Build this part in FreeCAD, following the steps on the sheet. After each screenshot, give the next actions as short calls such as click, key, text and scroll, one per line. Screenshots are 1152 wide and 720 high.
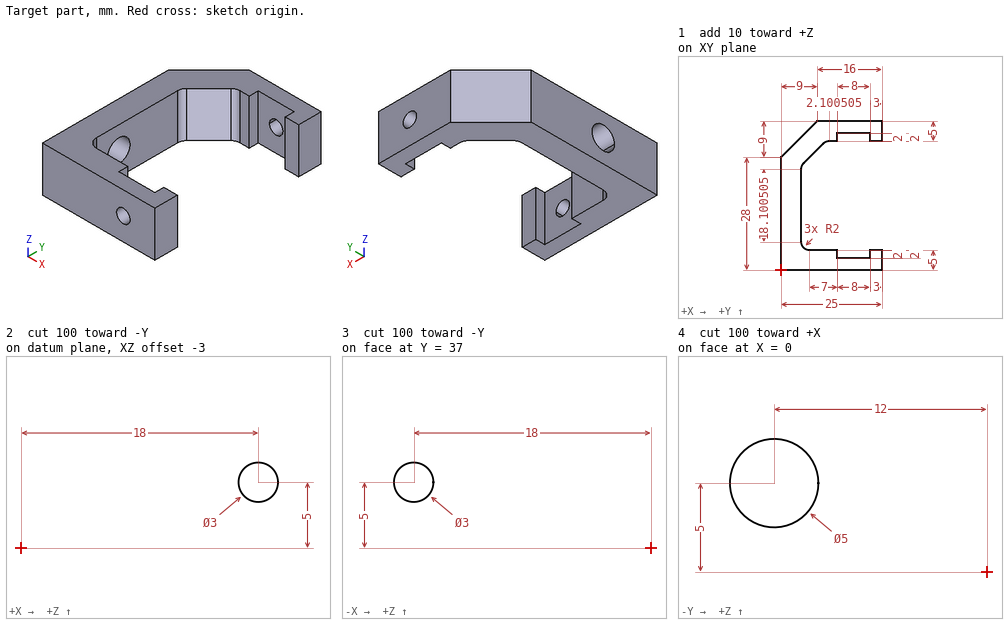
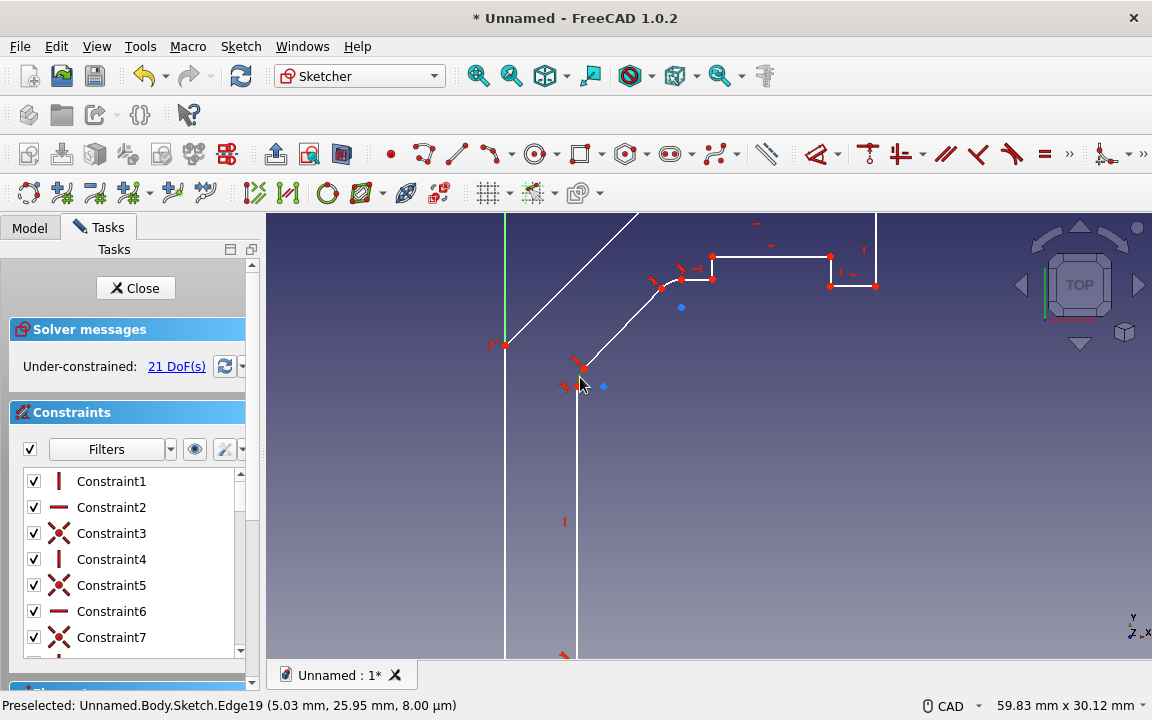
scroll(632, 324, up, 7)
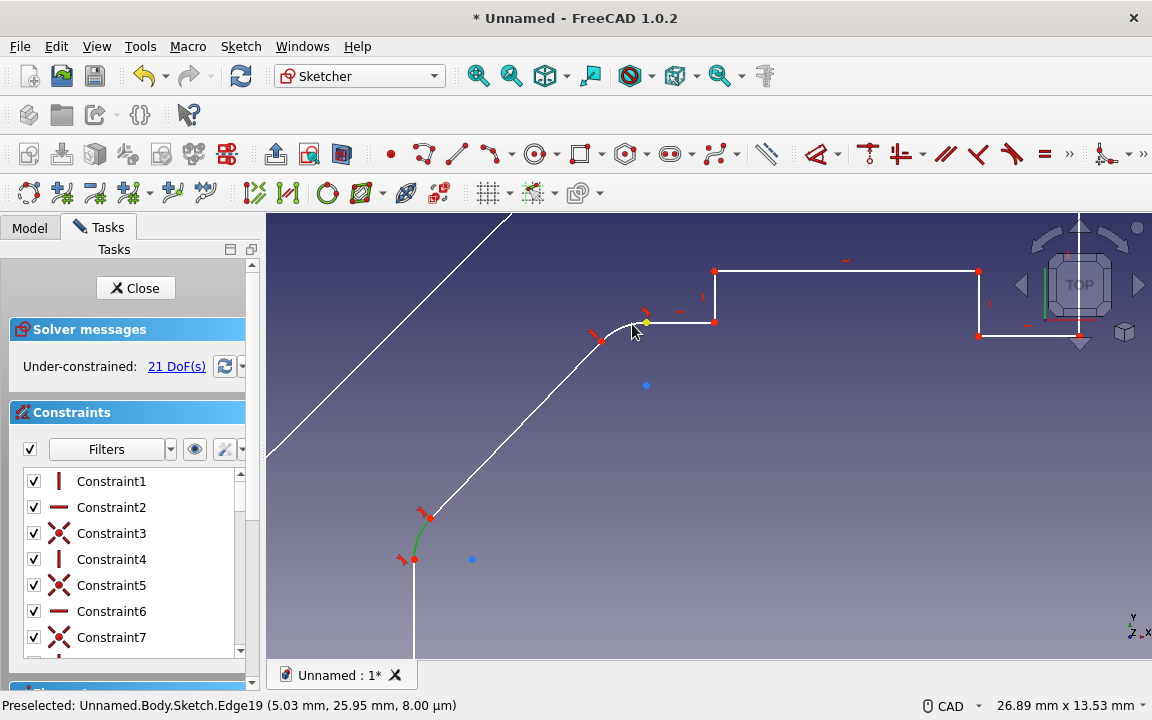
click(631, 324)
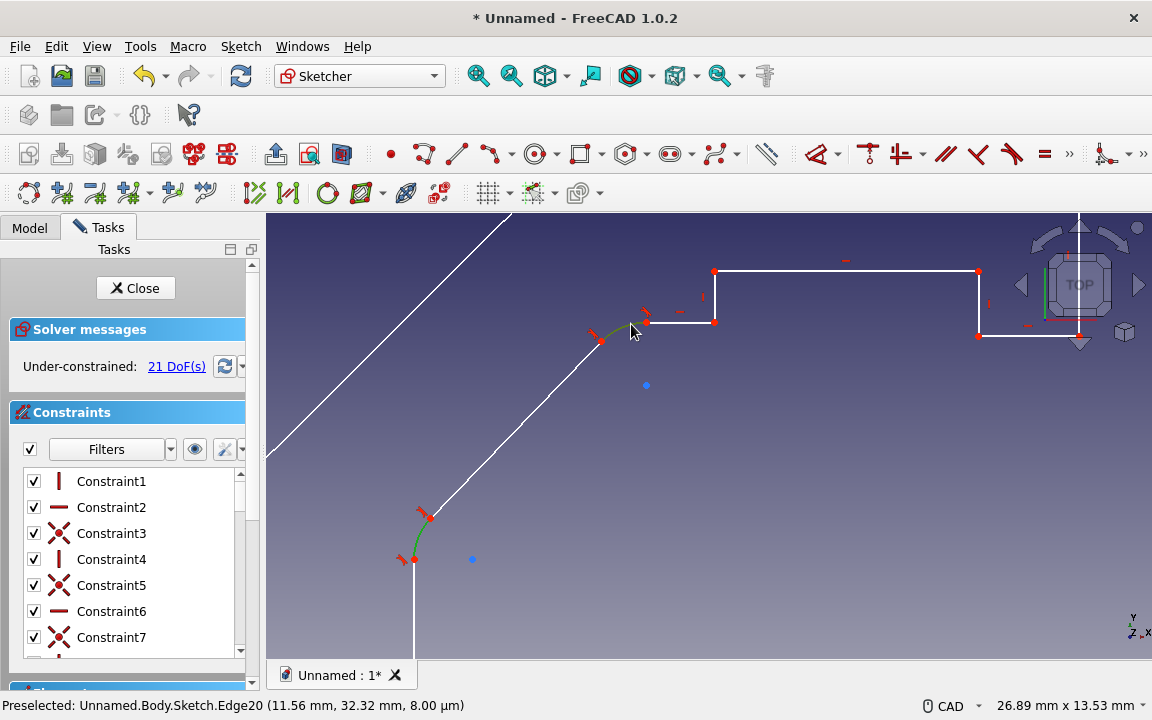
scroll(632, 324, down, 7)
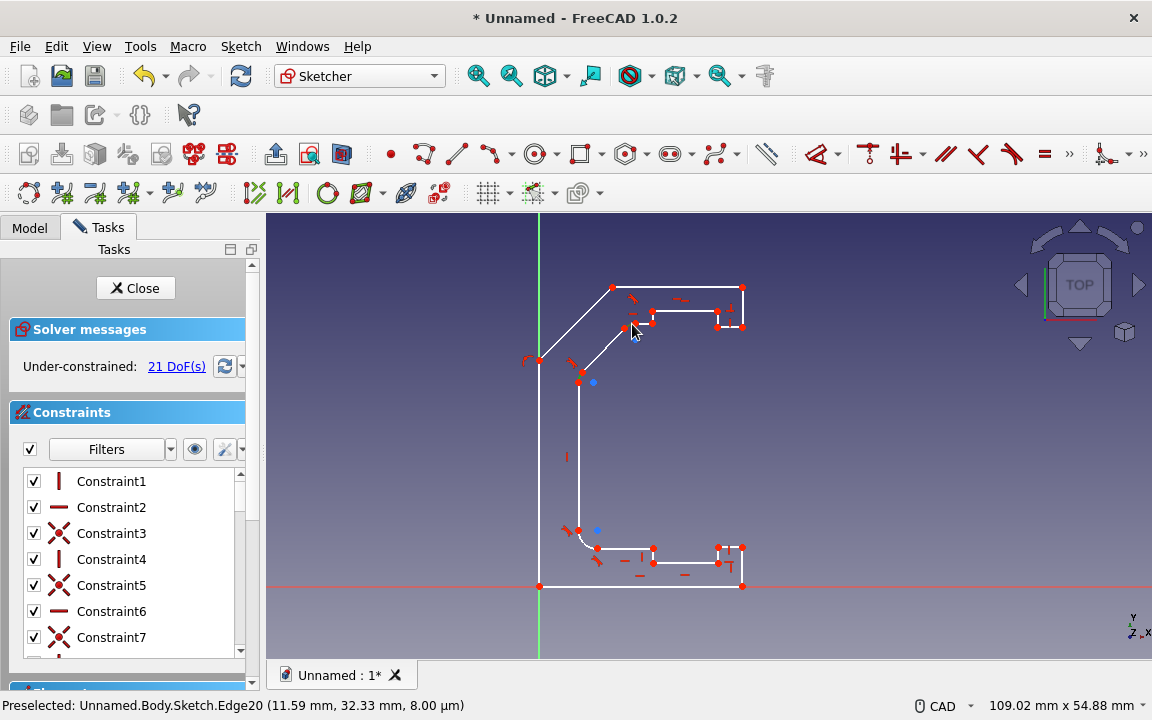
scroll(581, 539, up, 3)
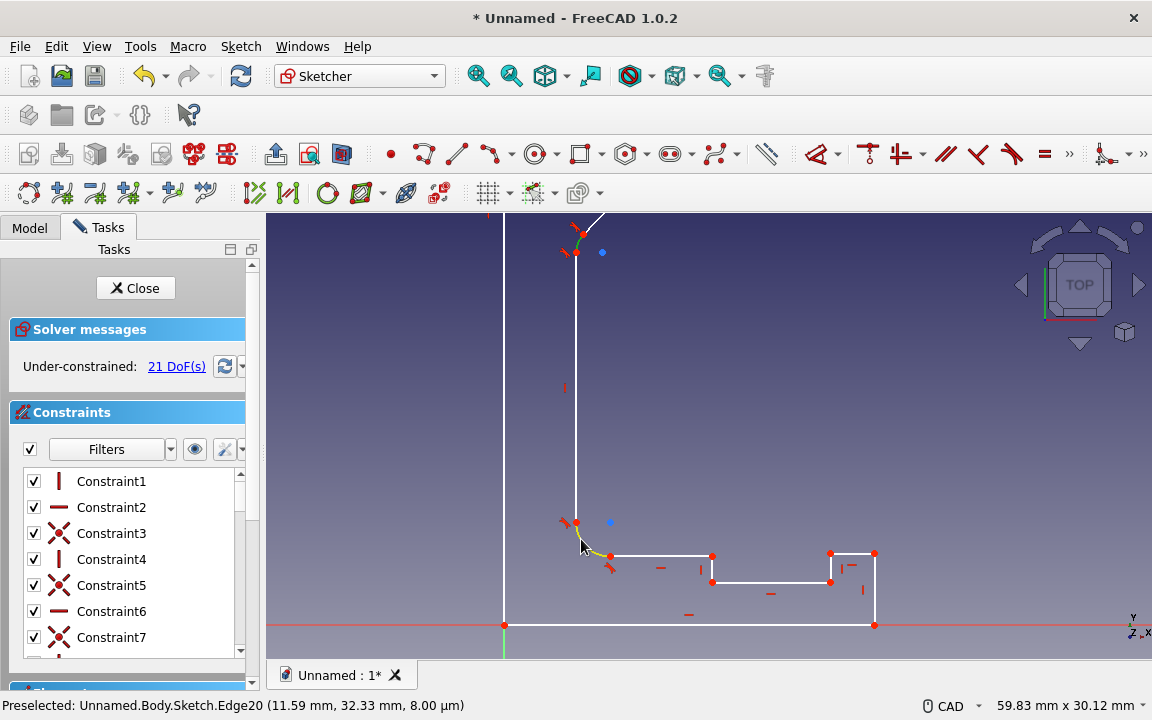
click(580, 538)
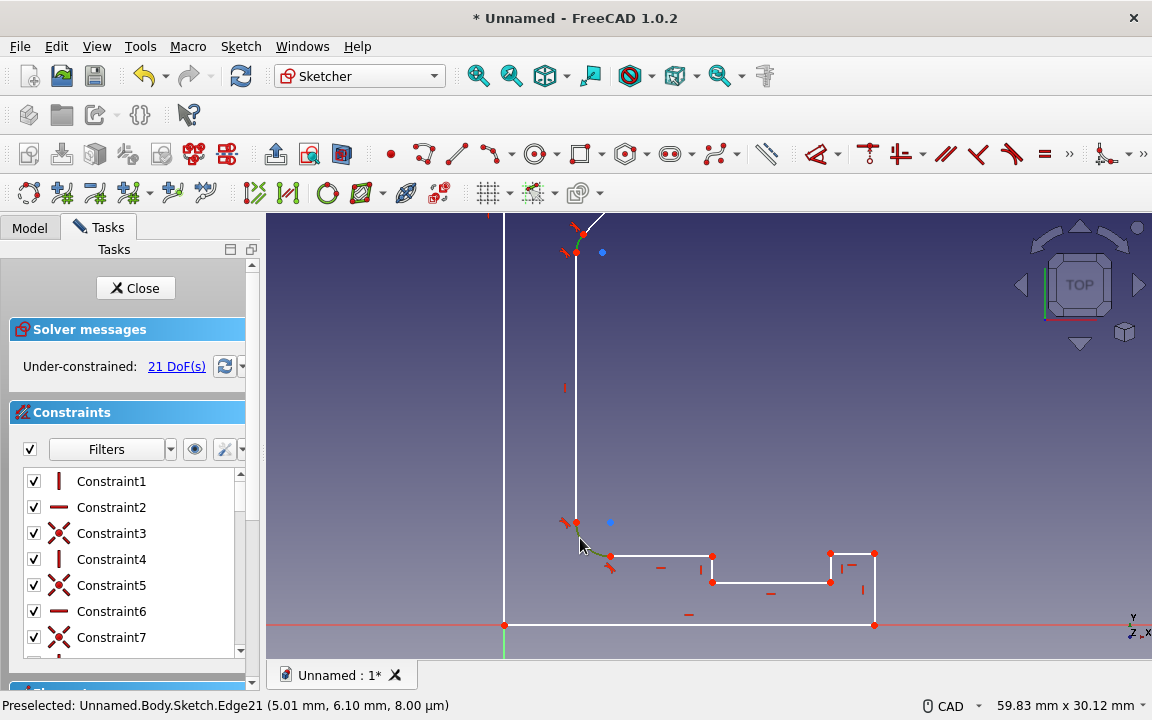
key(e)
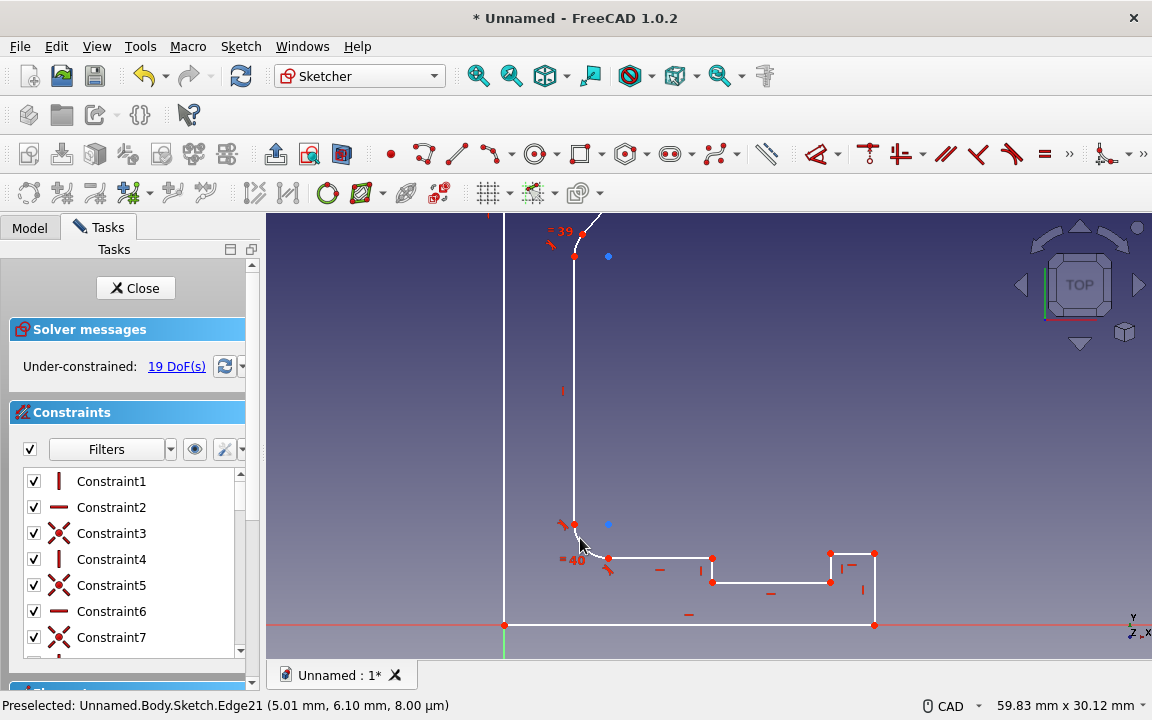
key(d)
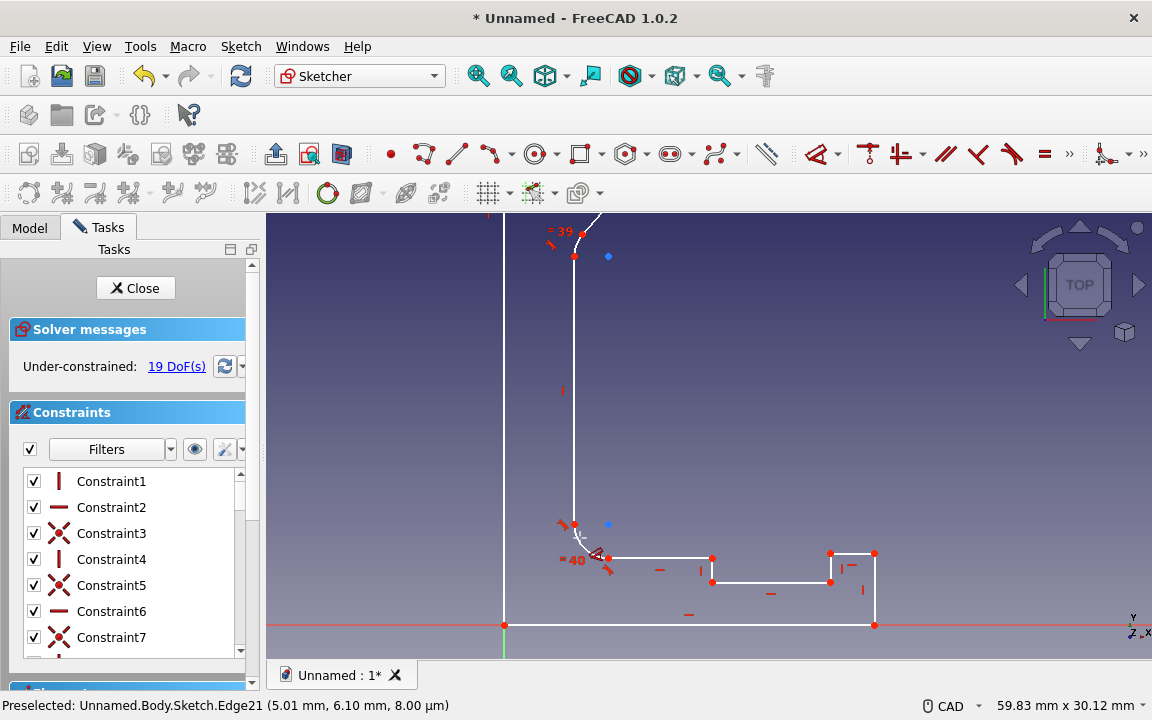
scroll(577, 245, up, 2)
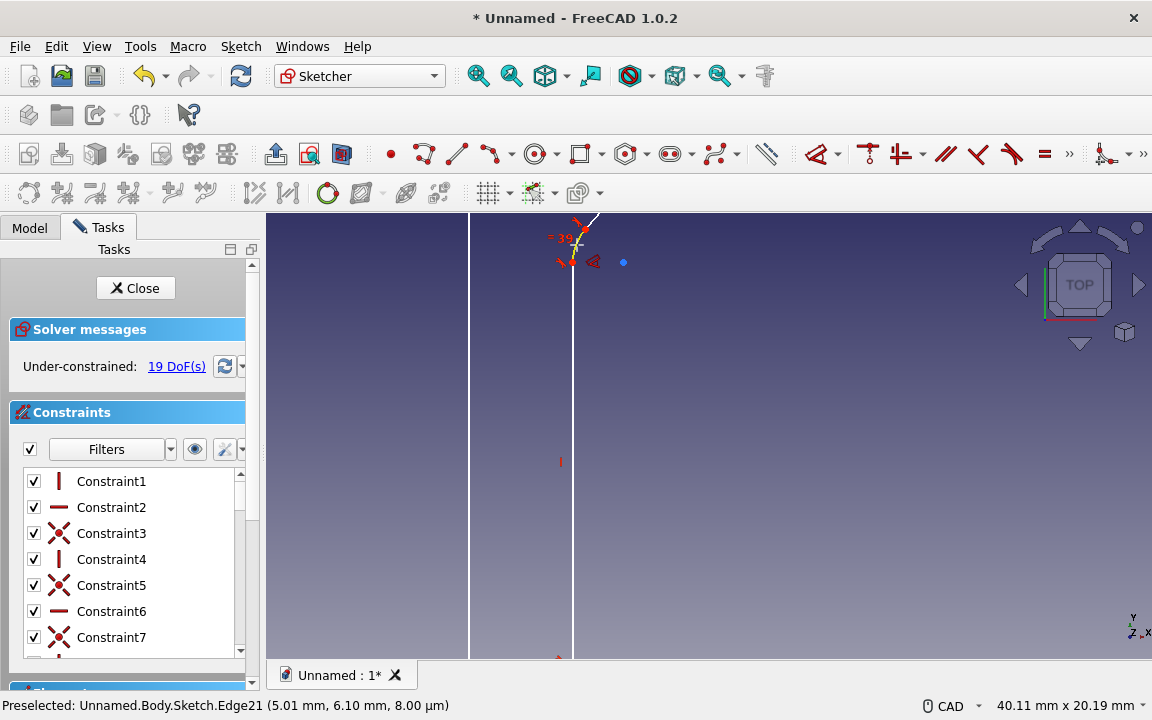
click(576, 245)
click(542, 275)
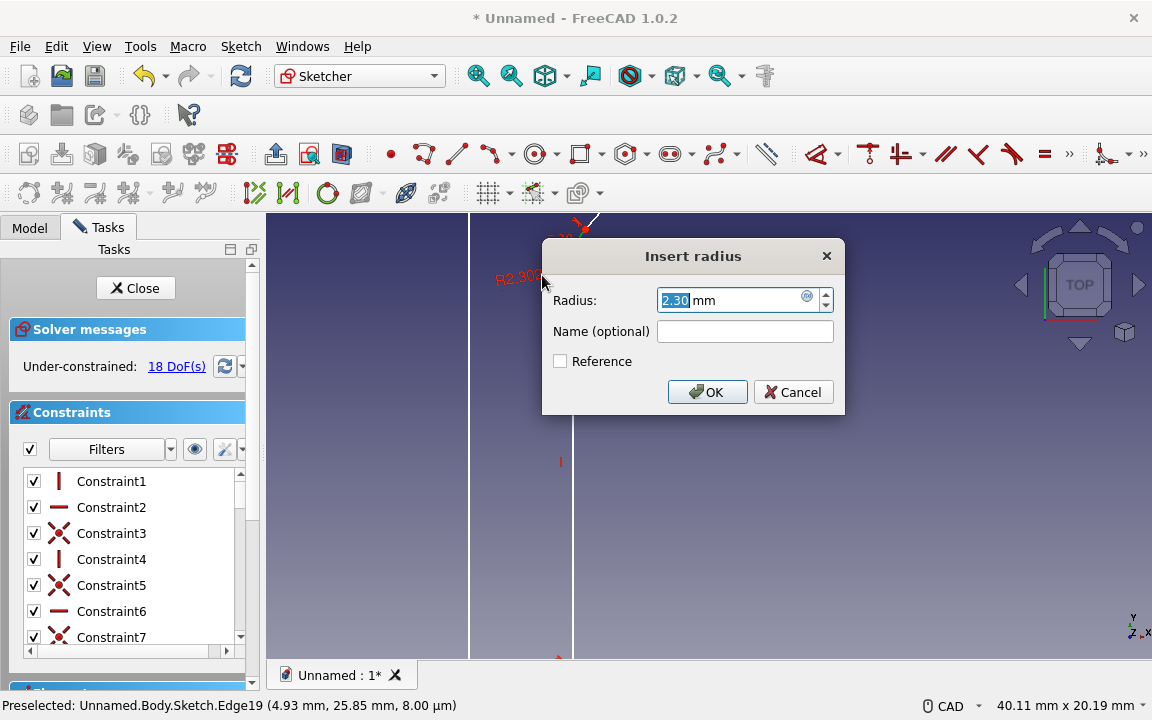
text(2)
key(Return)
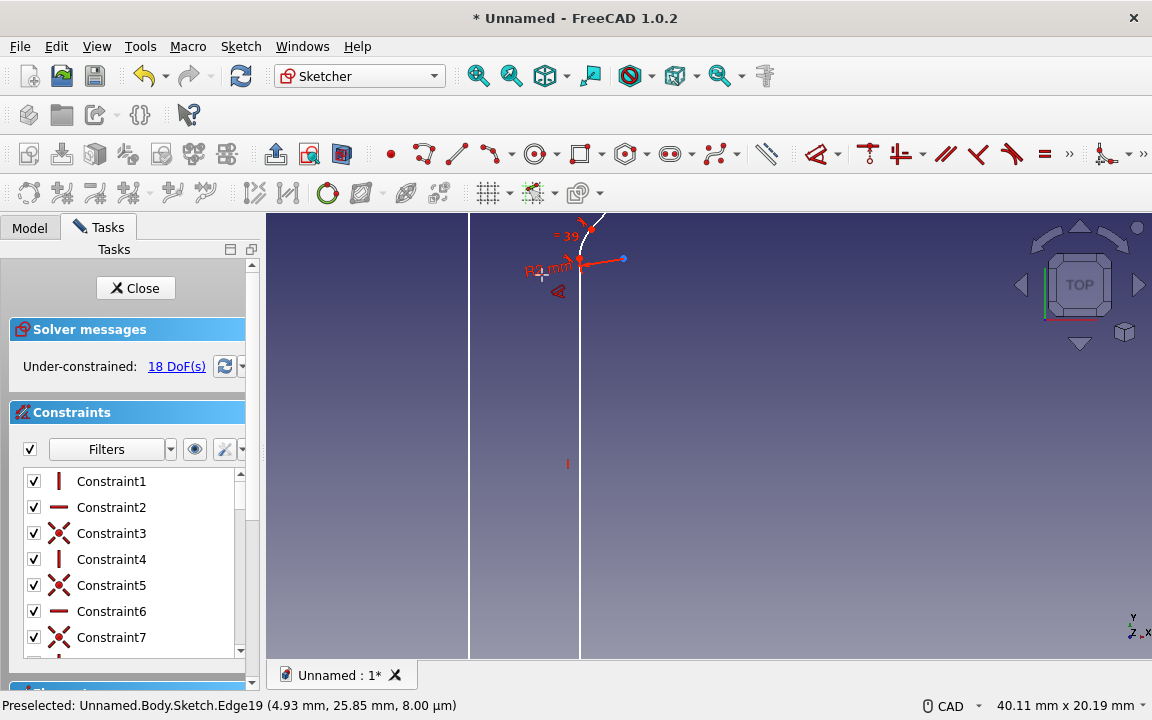
scroll(580, 455, down, 5)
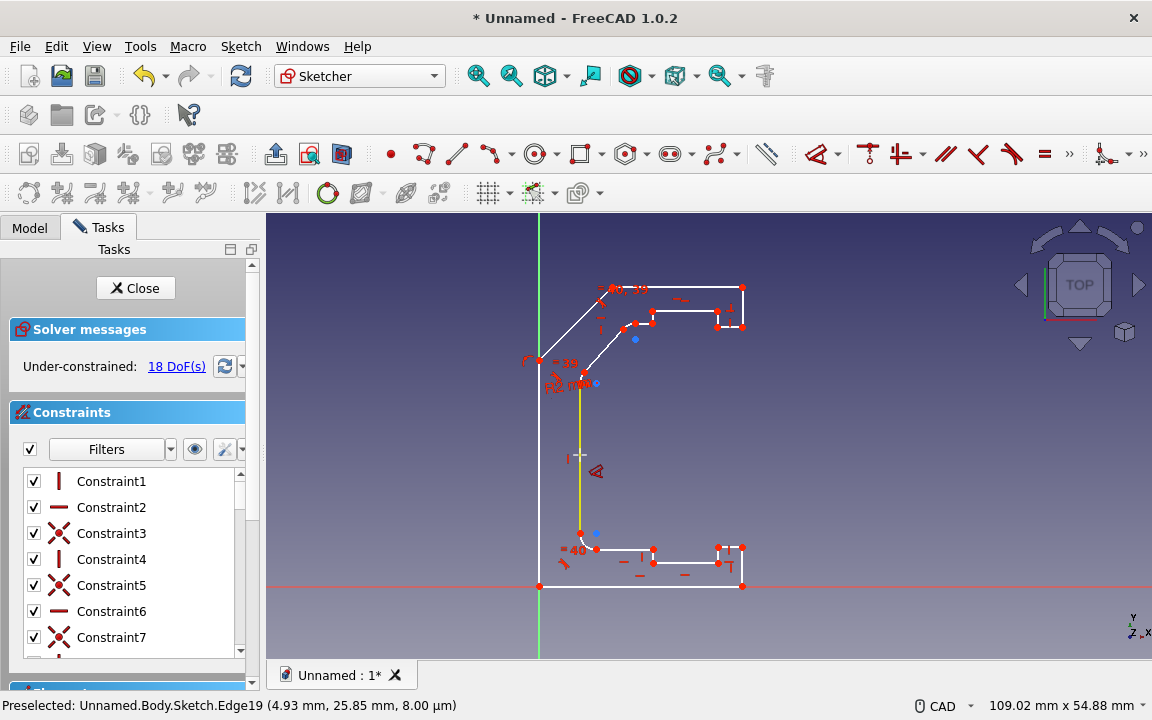
scroll(653, 320, up, 7)